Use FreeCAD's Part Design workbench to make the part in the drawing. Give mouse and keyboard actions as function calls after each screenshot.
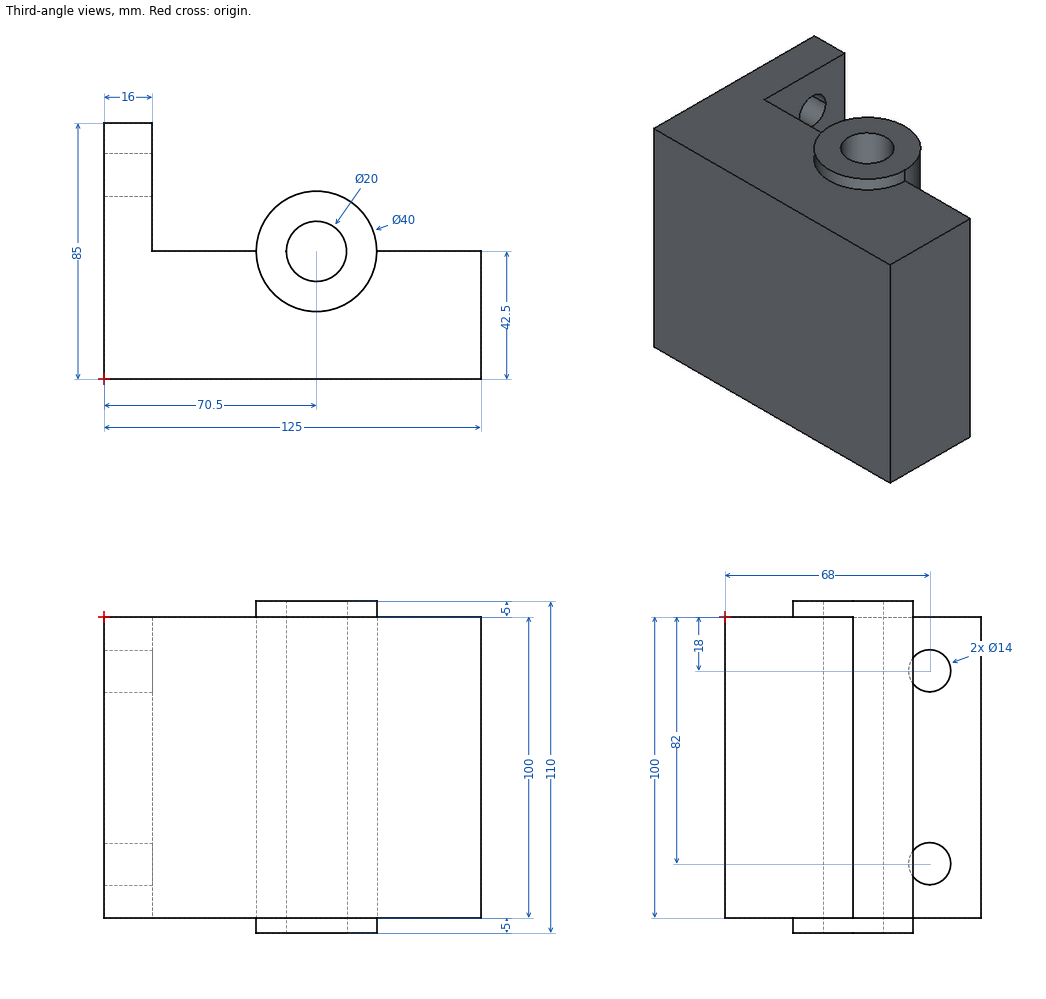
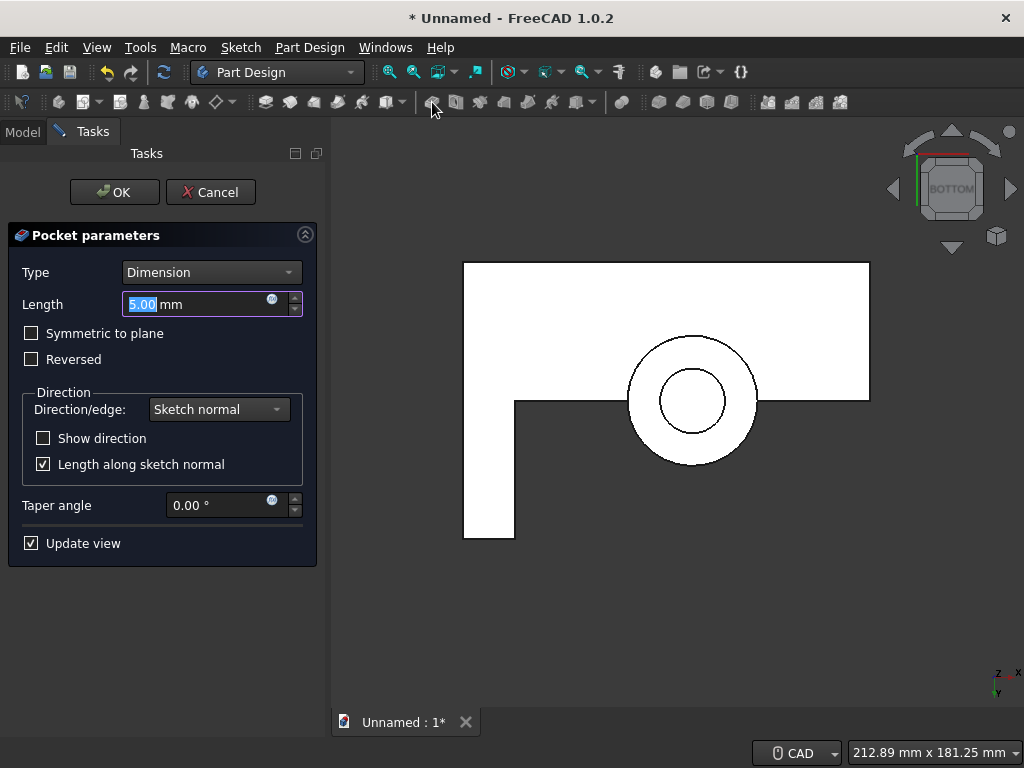
text(110)
key(Tab)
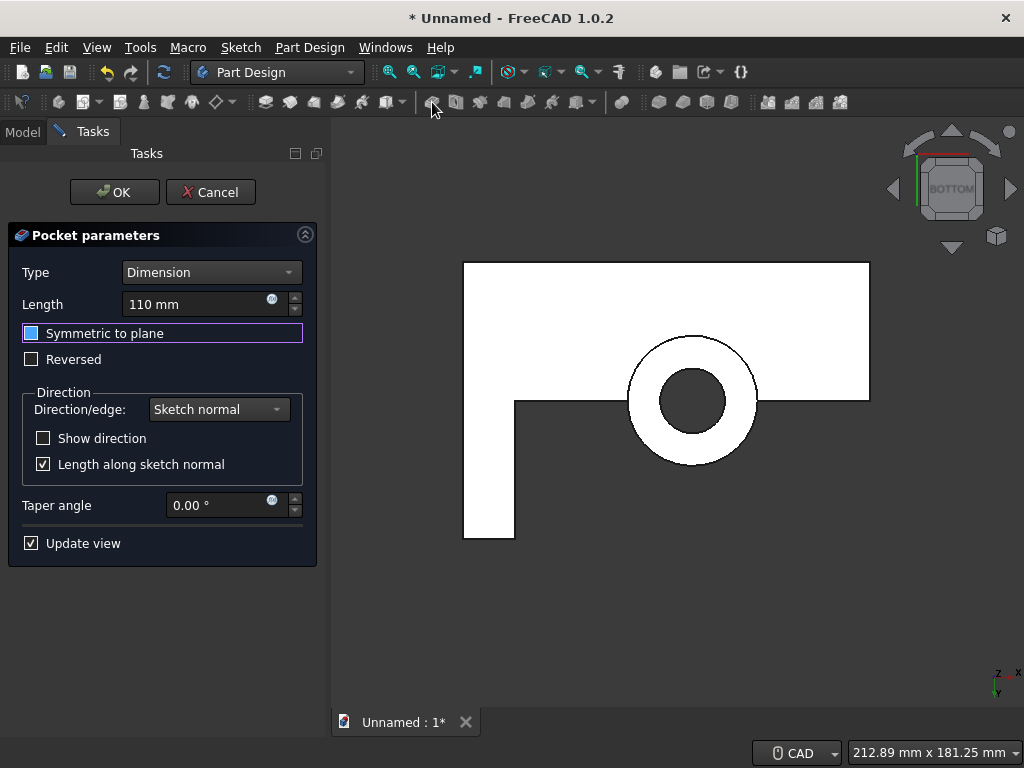
click(115, 192)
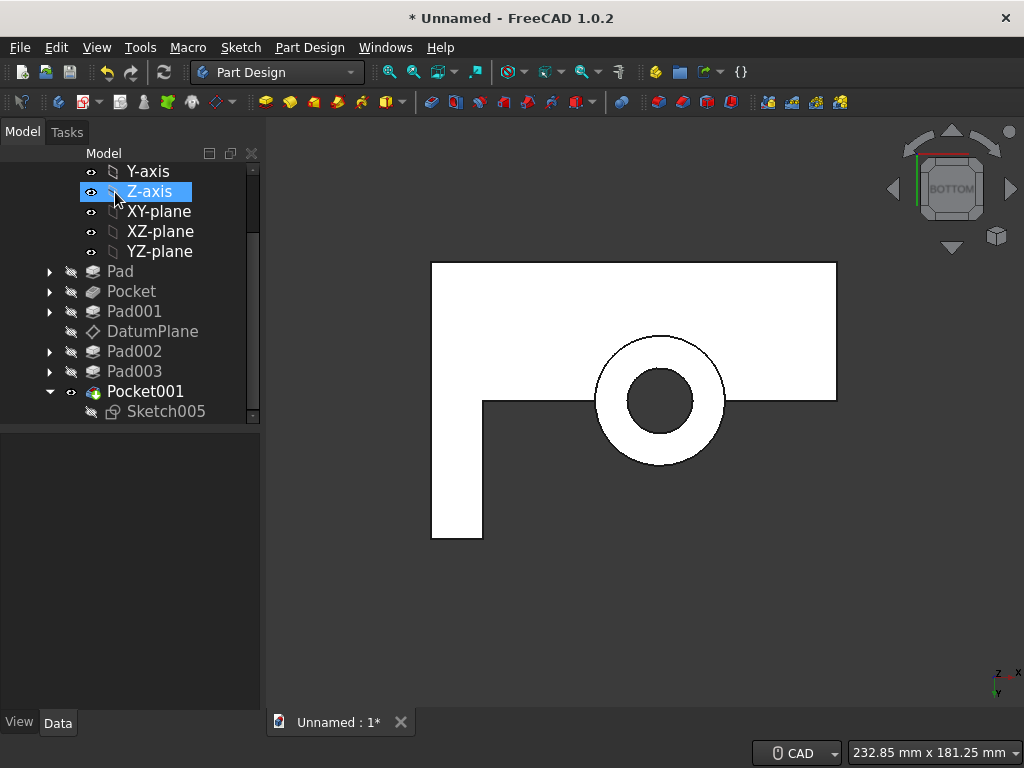
key(0)